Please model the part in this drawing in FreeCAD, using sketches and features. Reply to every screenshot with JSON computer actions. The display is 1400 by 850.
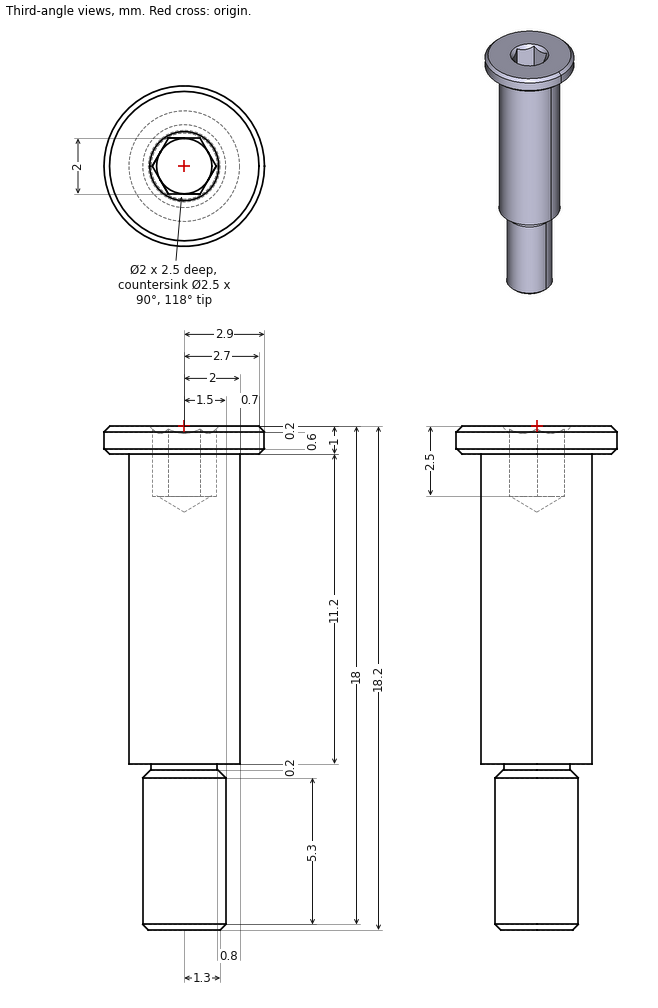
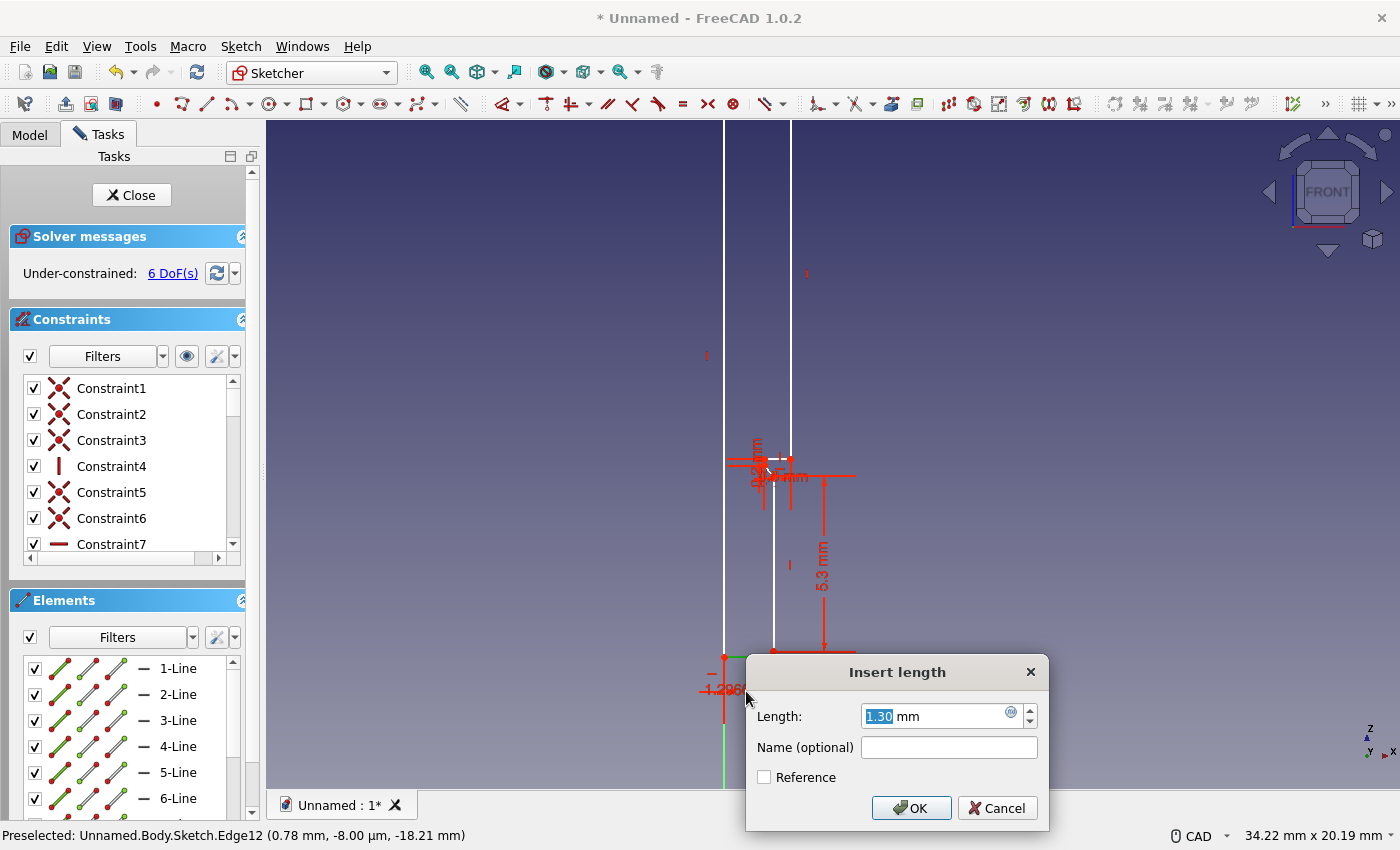
{"action": "type", "text": "1.3"}
{"action": "key", "text": "Return"}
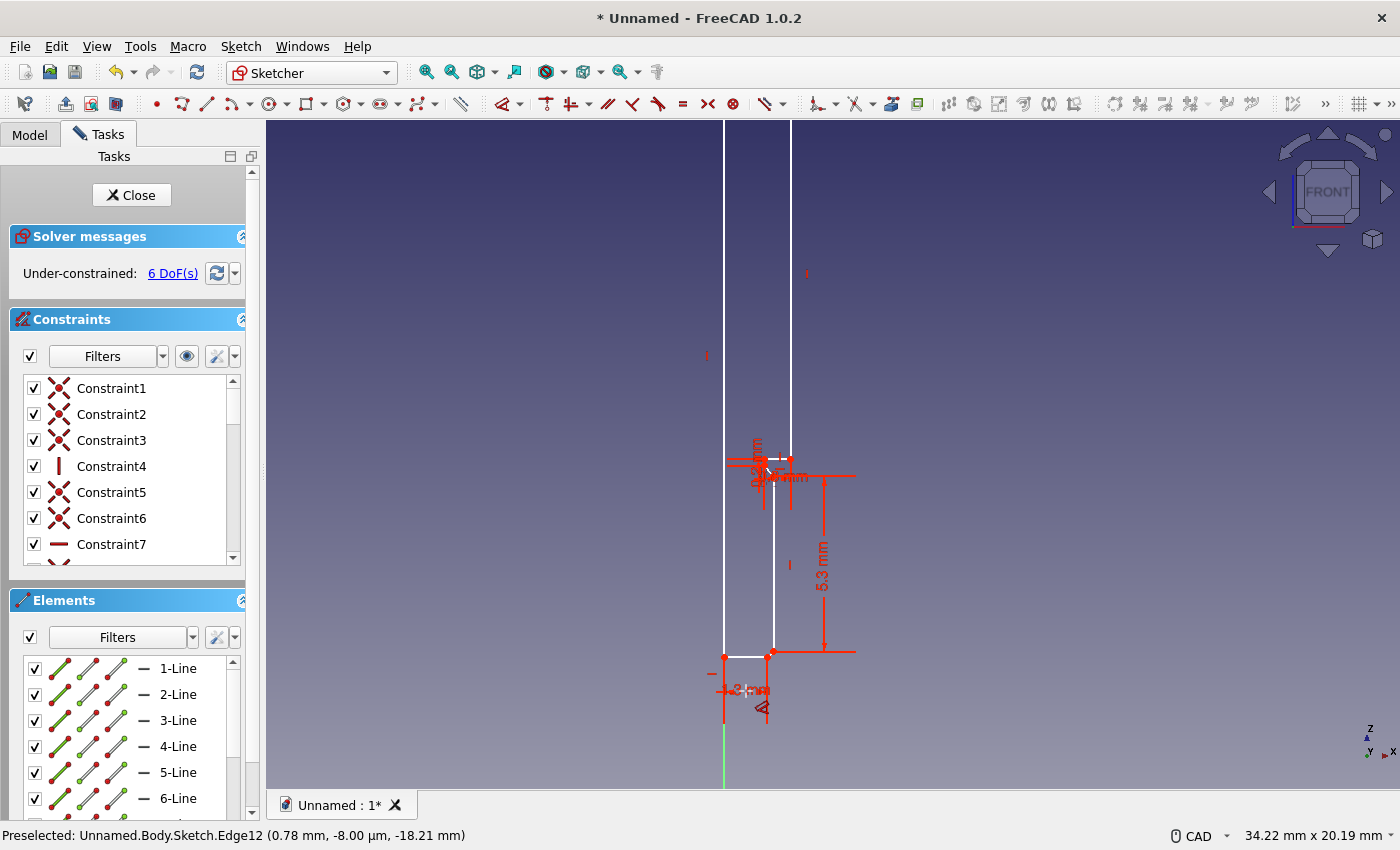
{"action": "scroll", "coordinate": [774, 652], "scroll_direction": "up", "scroll_amount": 2}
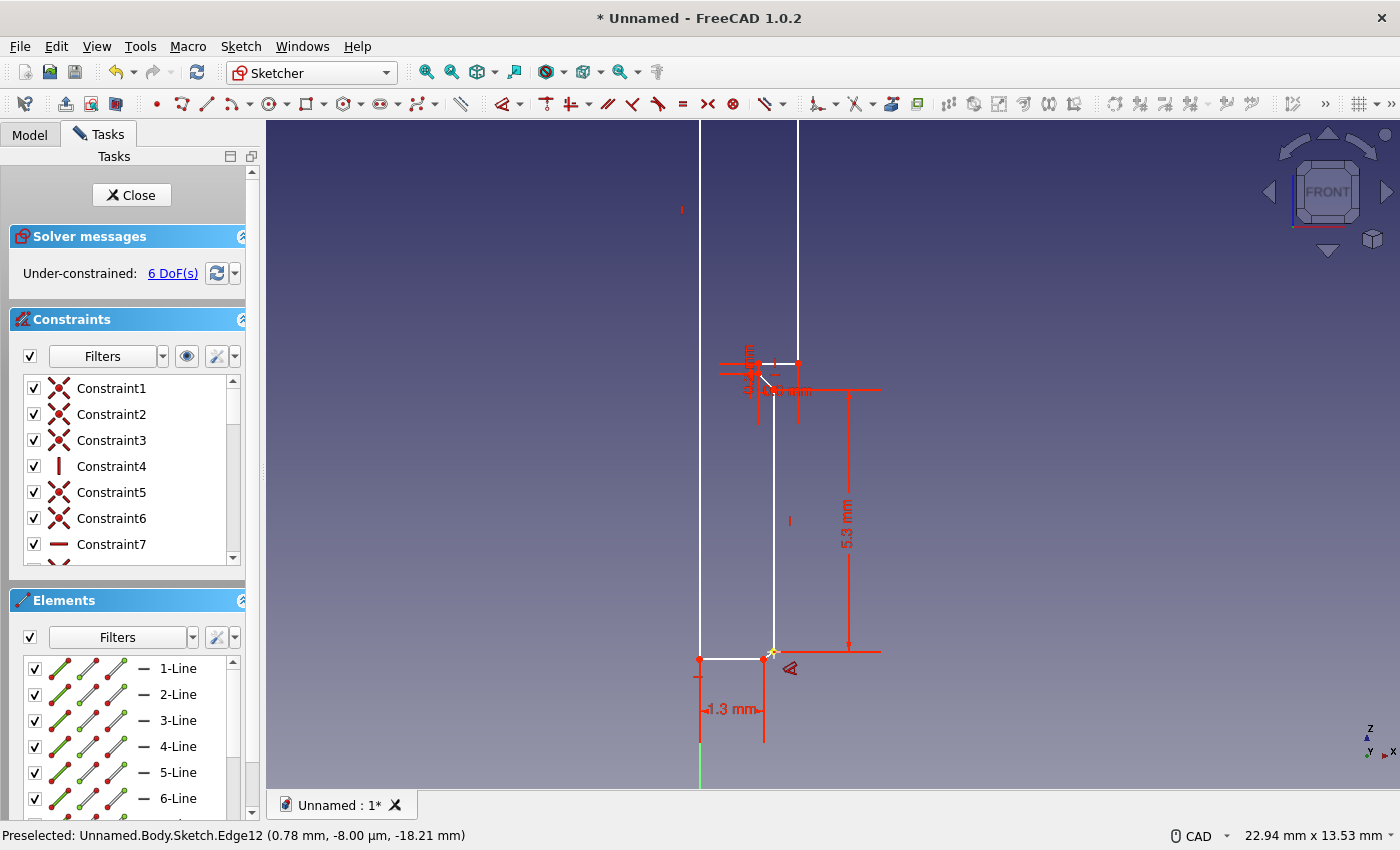
{"action": "left_click", "coordinate": [774, 652]}
{"action": "left_click", "coordinate": [666, 400]}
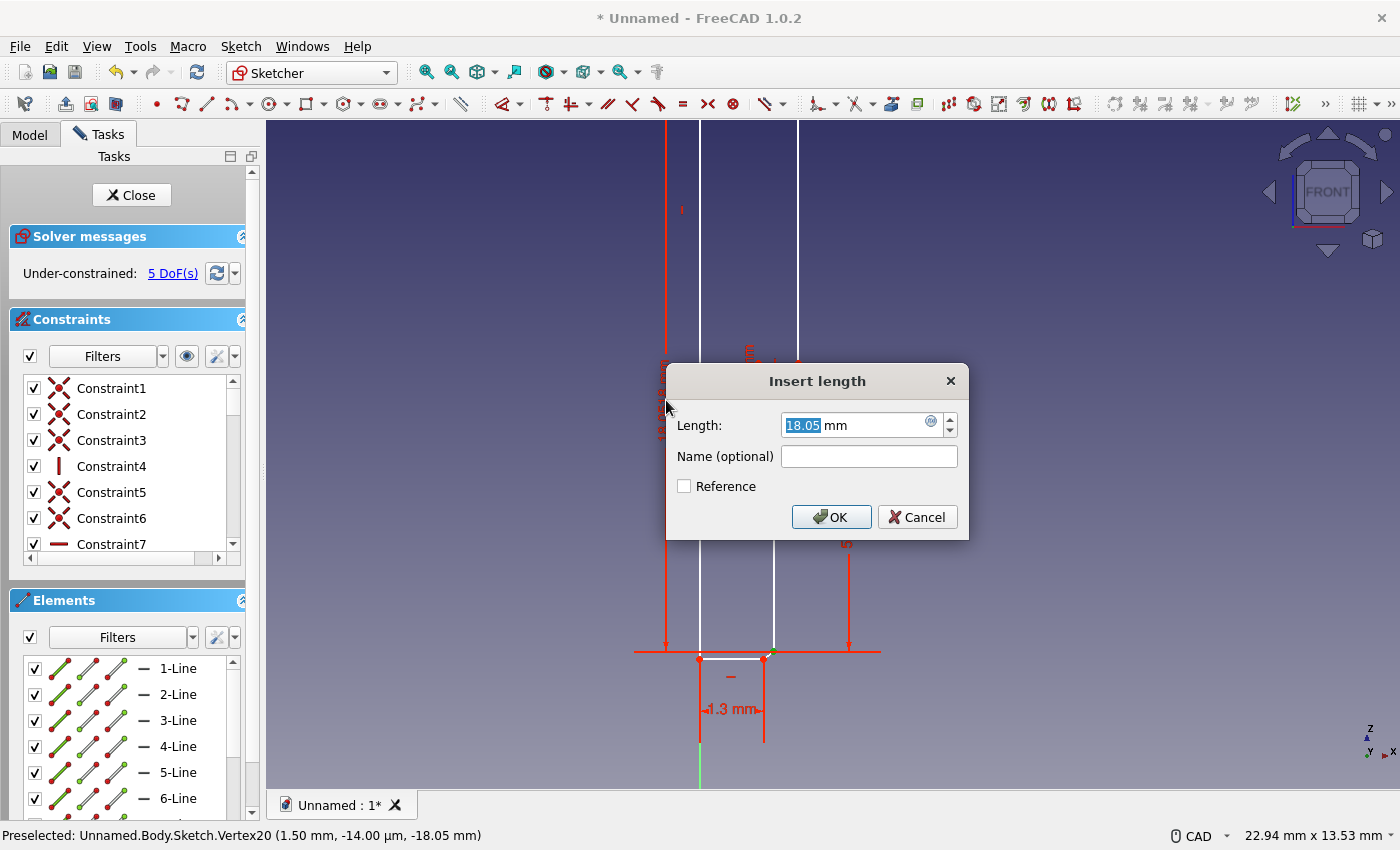
{"action": "type", "text": "18"}
{"action": "key", "text": "Return"}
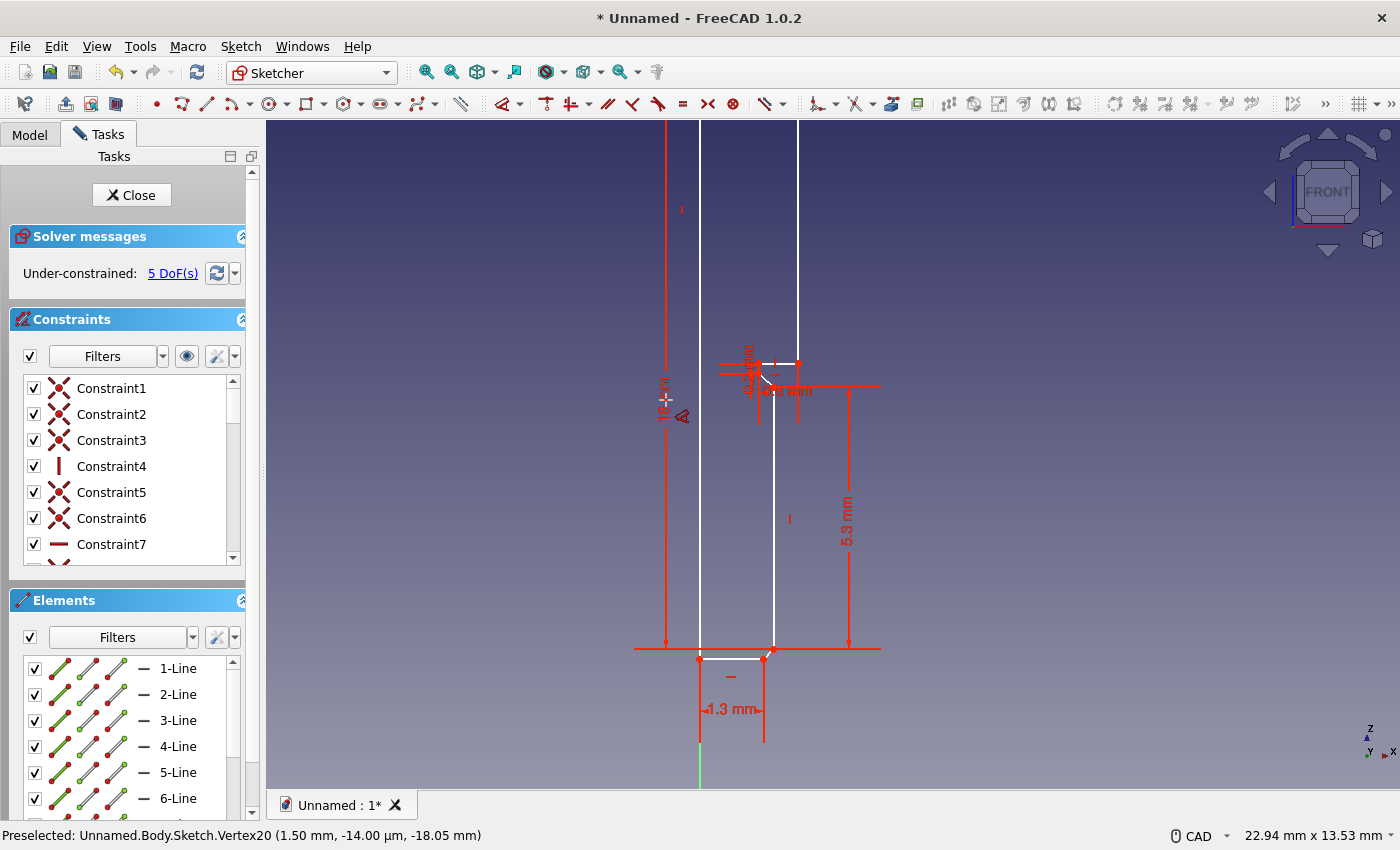
{"action": "left_click", "coordinate": [798, 197]}
{"action": "left_click", "coordinate": [832, 256]}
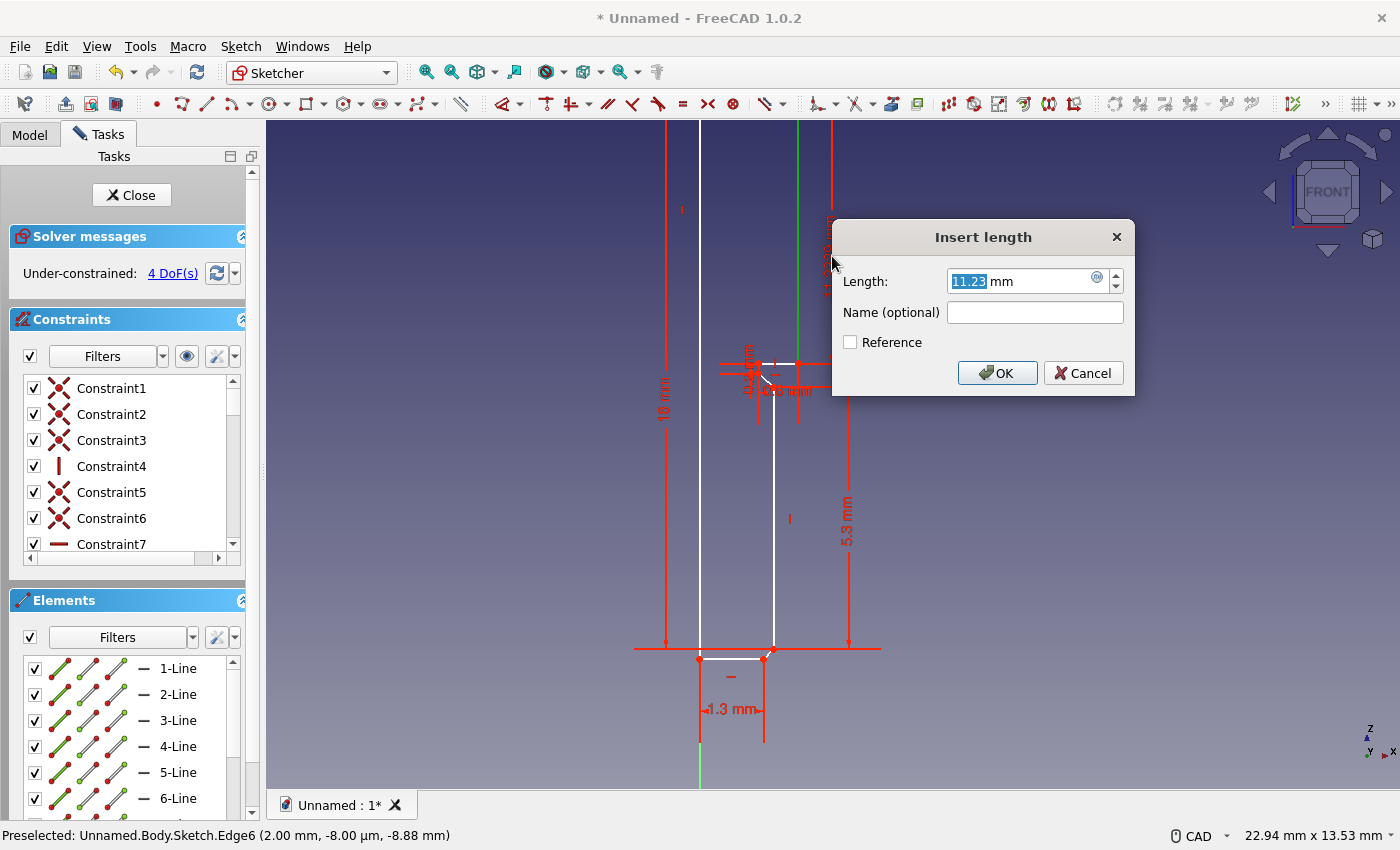
{"action": "type", "text": "11.2"}
{"action": "key", "text": "Return"}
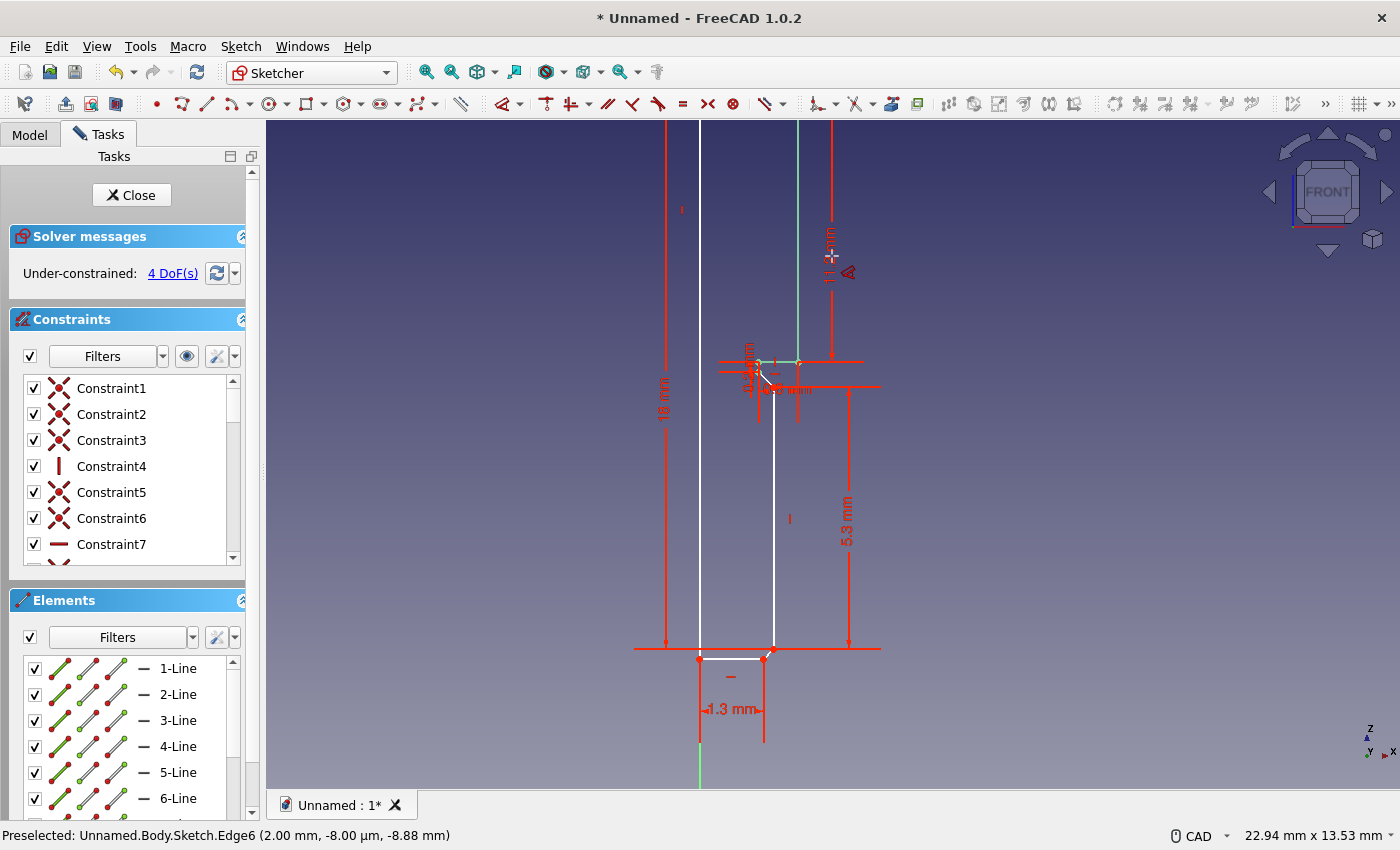
{"action": "left_click", "coordinate": [700, 389]}
{"action": "left_click", "coordinate": [666, 286]}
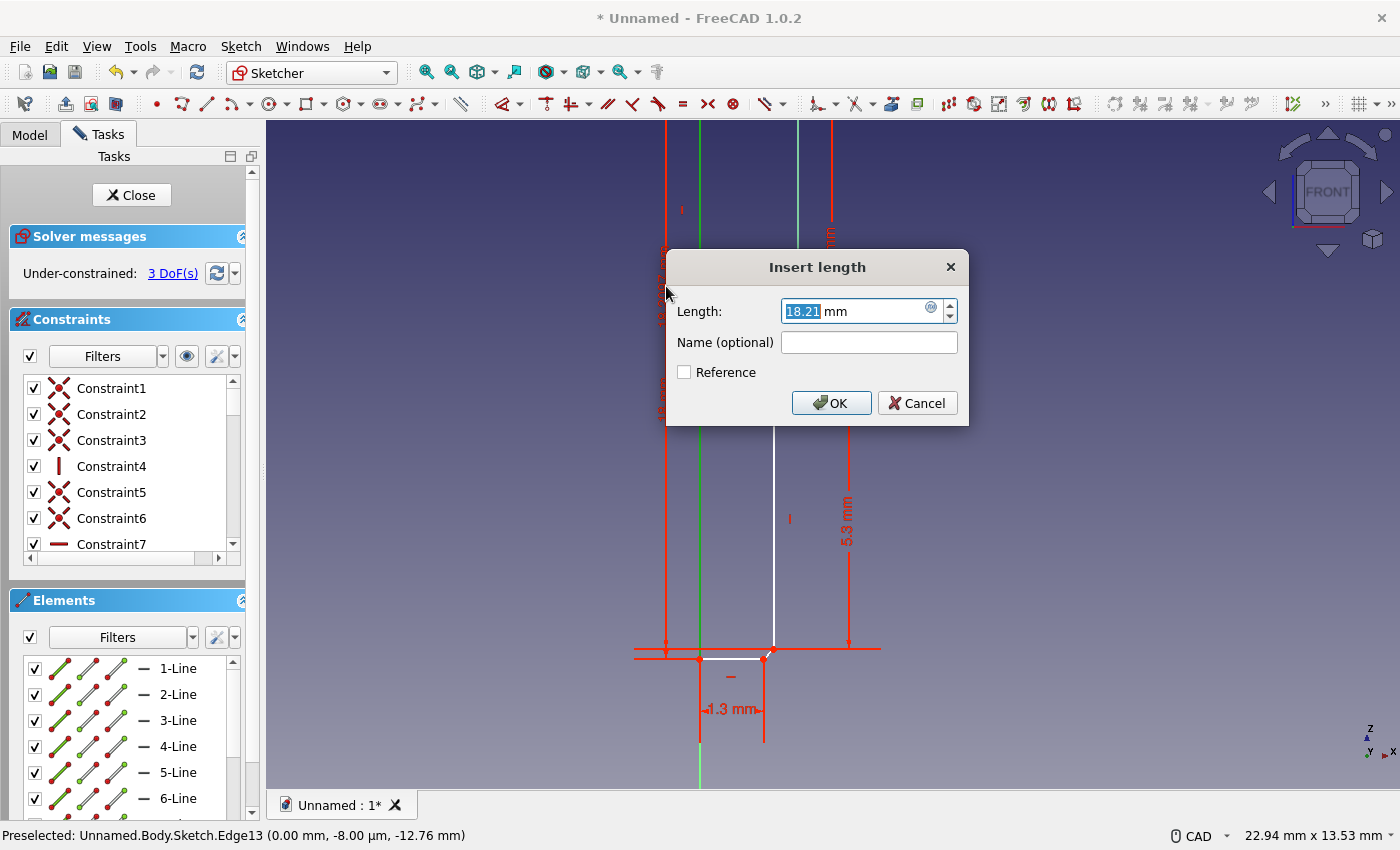
{"action": "type", "text": "18.2"}
{"action": "key", "text": "Return"}